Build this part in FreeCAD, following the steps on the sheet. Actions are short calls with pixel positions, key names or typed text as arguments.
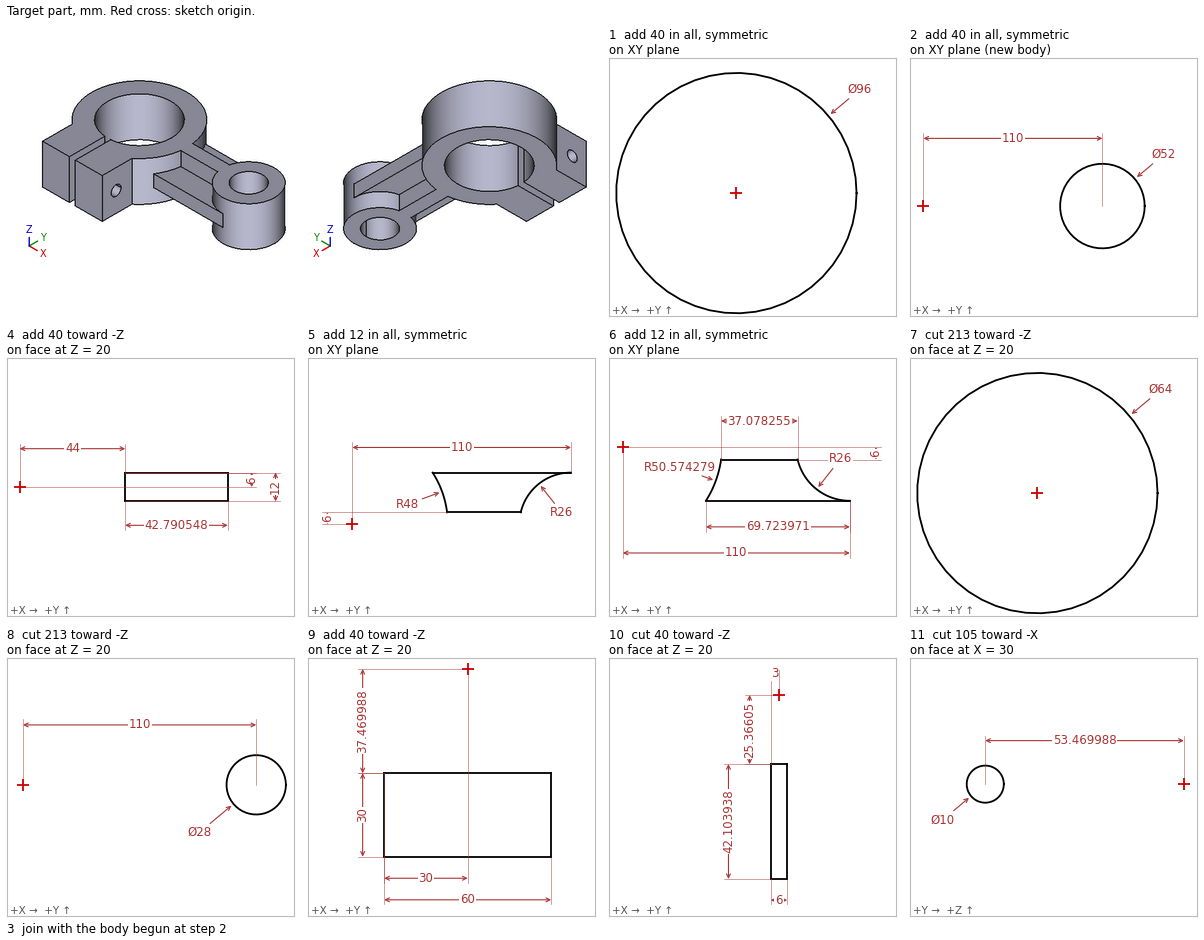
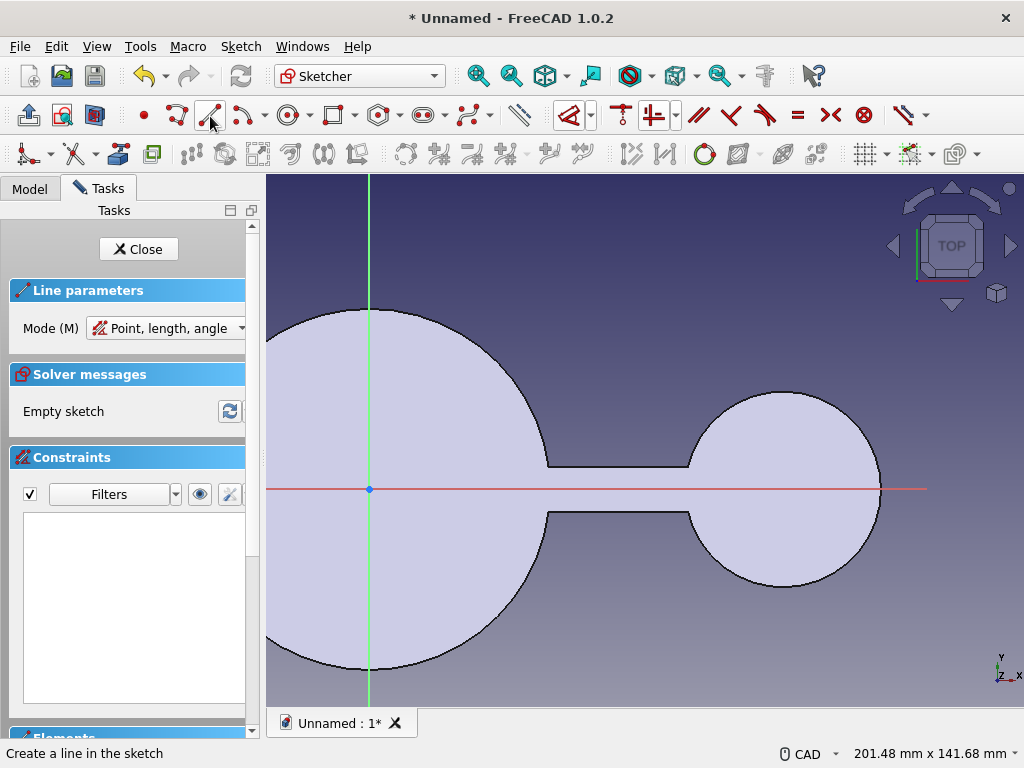
click(783, 392)
click(521, 392)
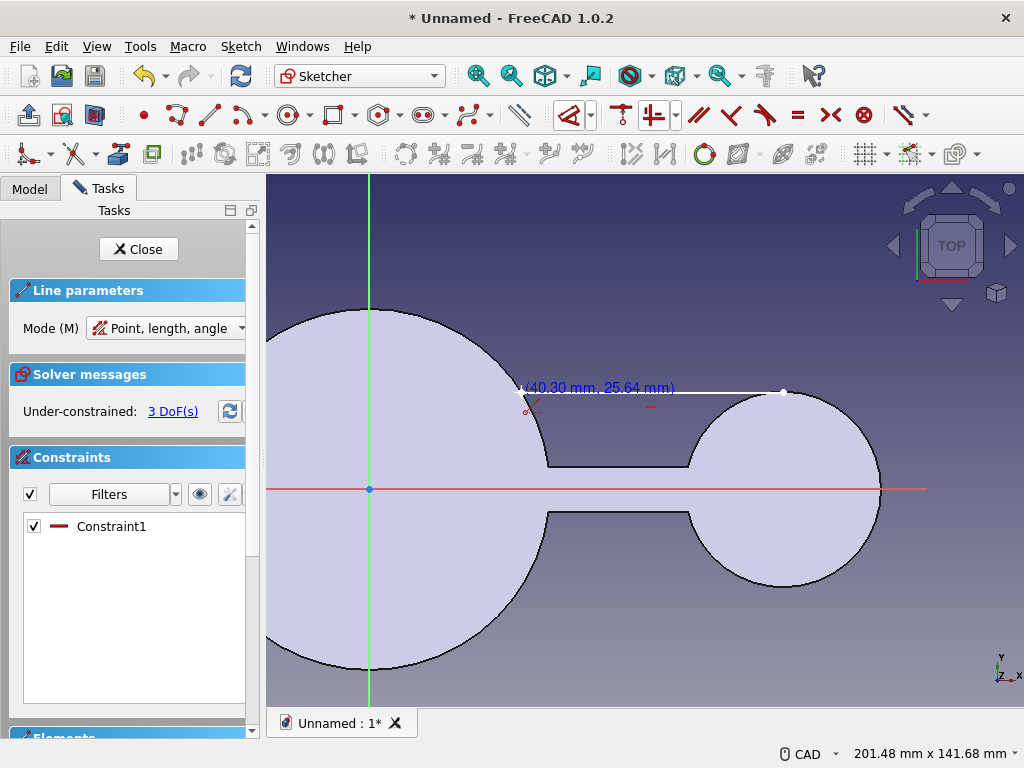
click(549, 467)
click(688, 467)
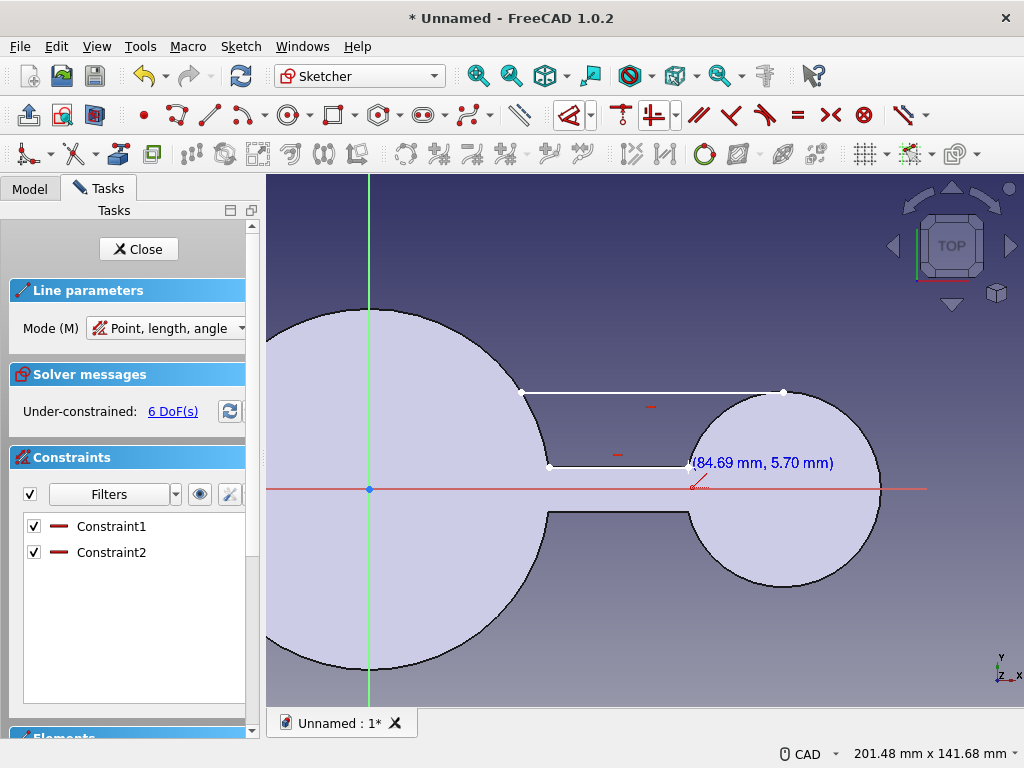
key(g)
key(3)
key(a)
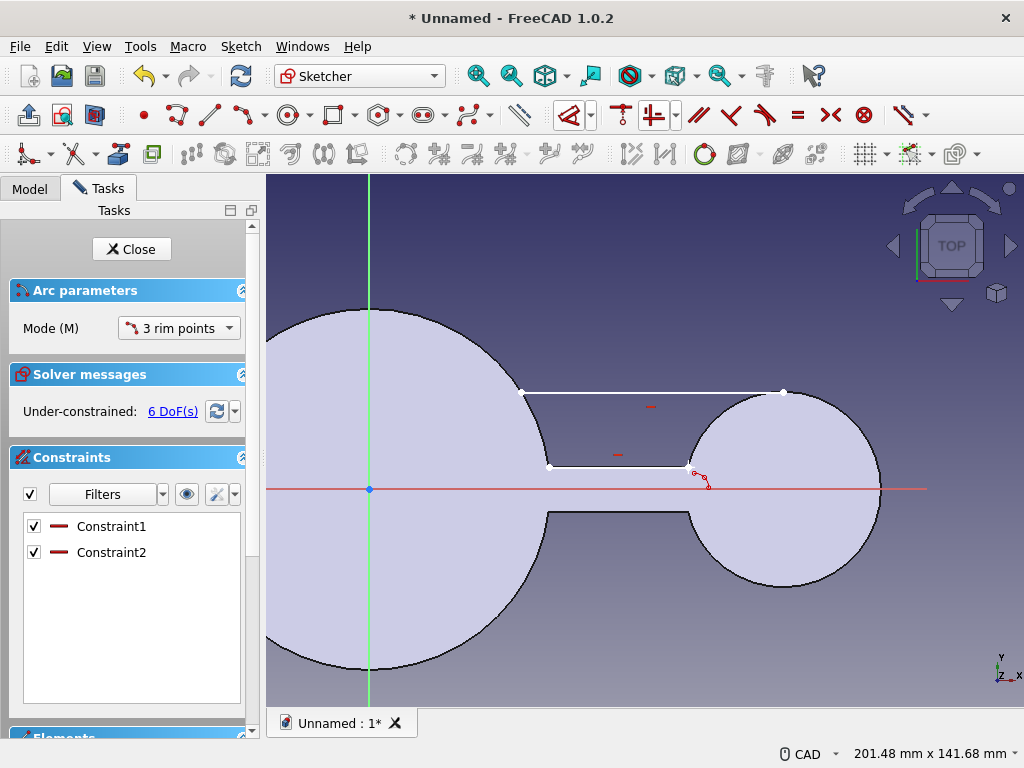
click(521, 393)
click(549, 468)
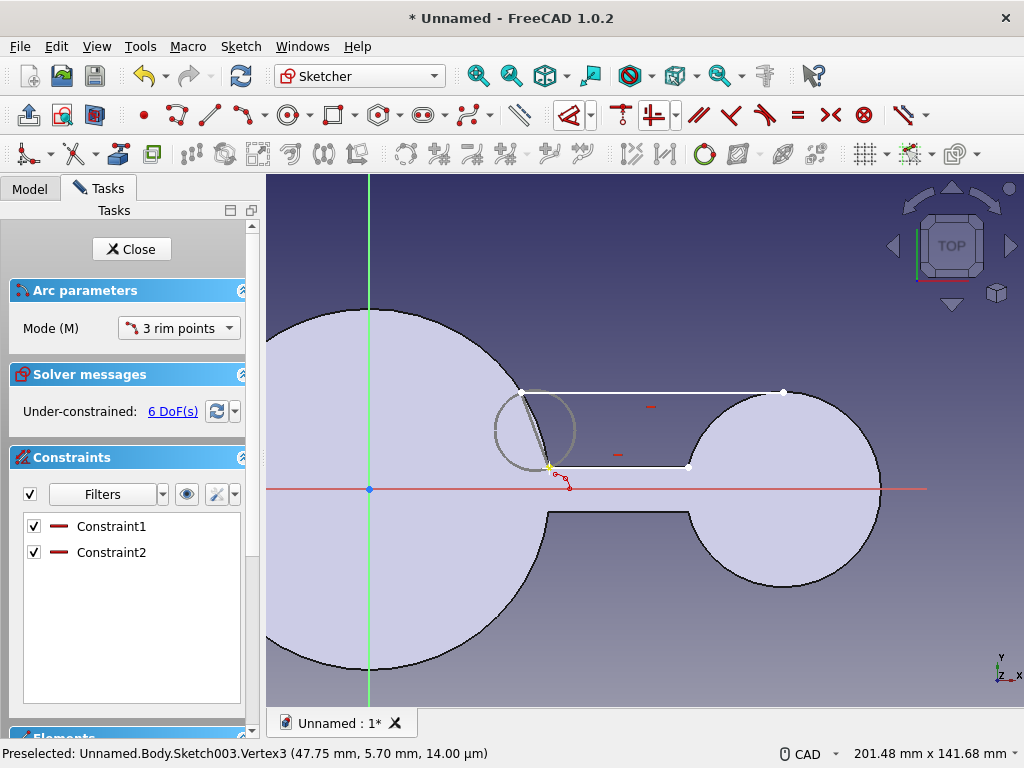
scroll(539, 428, up, 7)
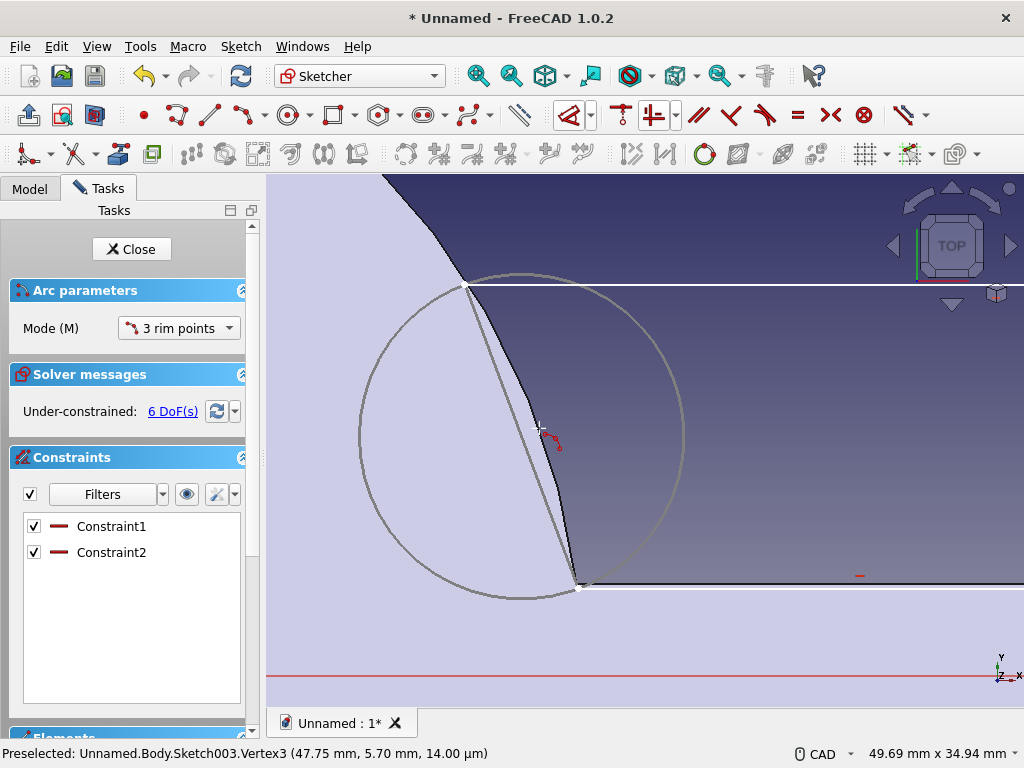
click(538, 425)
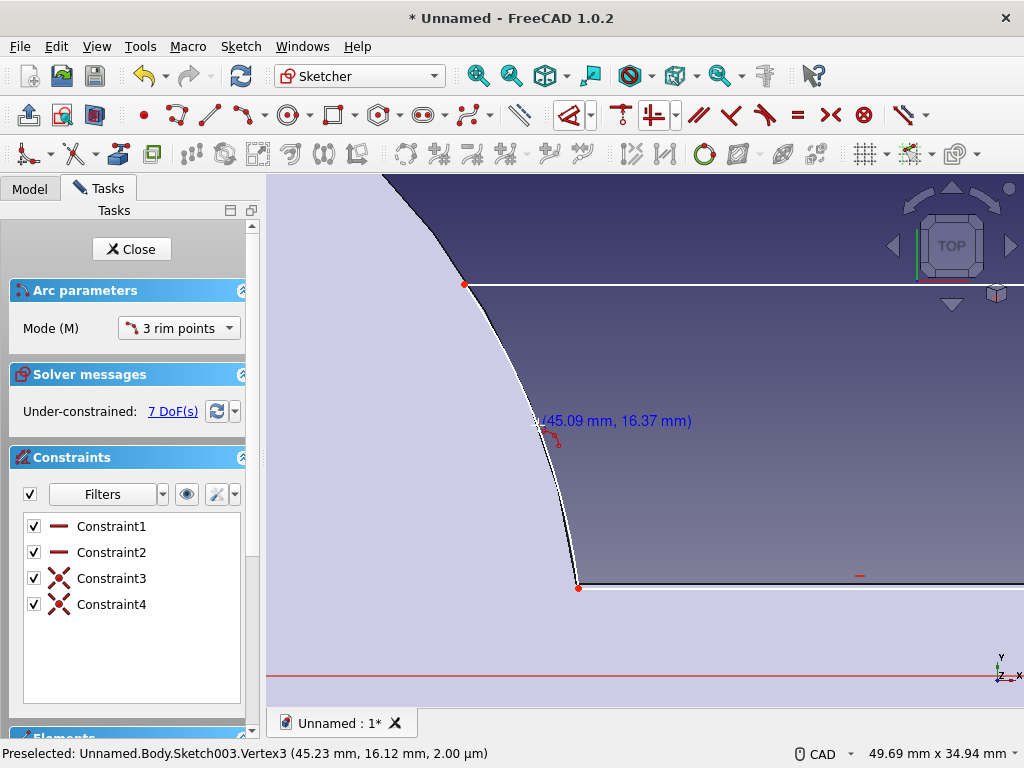
scroll(540, 428, down, 7)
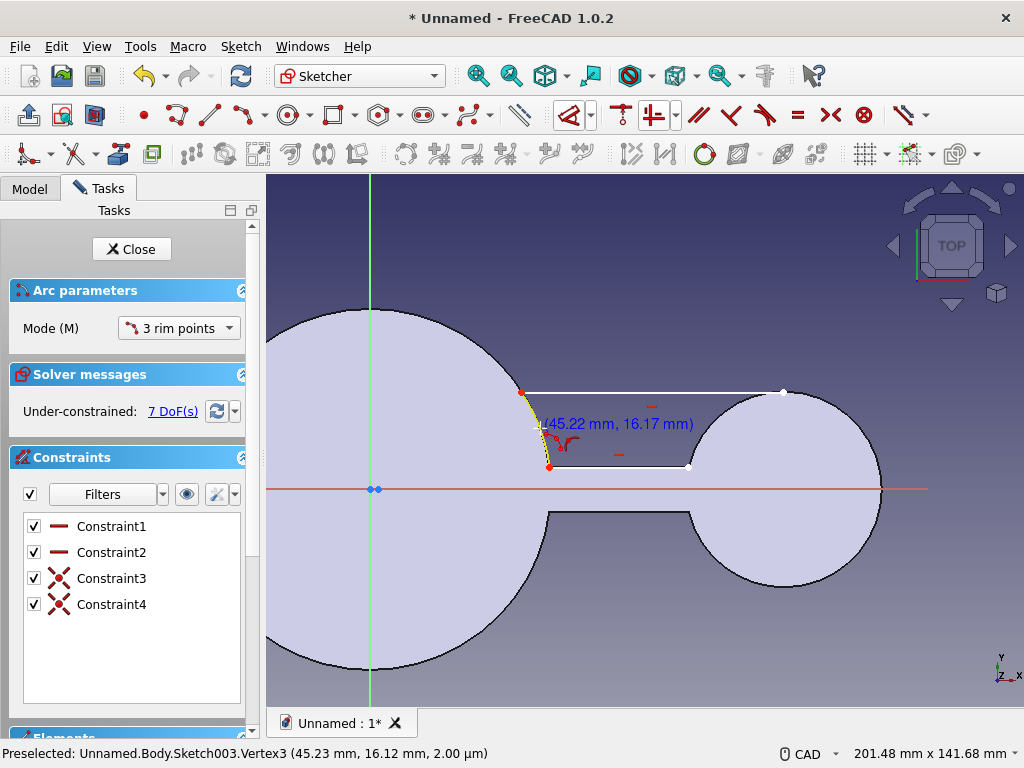
click(689, 468)
click(784, 393)
click(723, 413)
key(Escape)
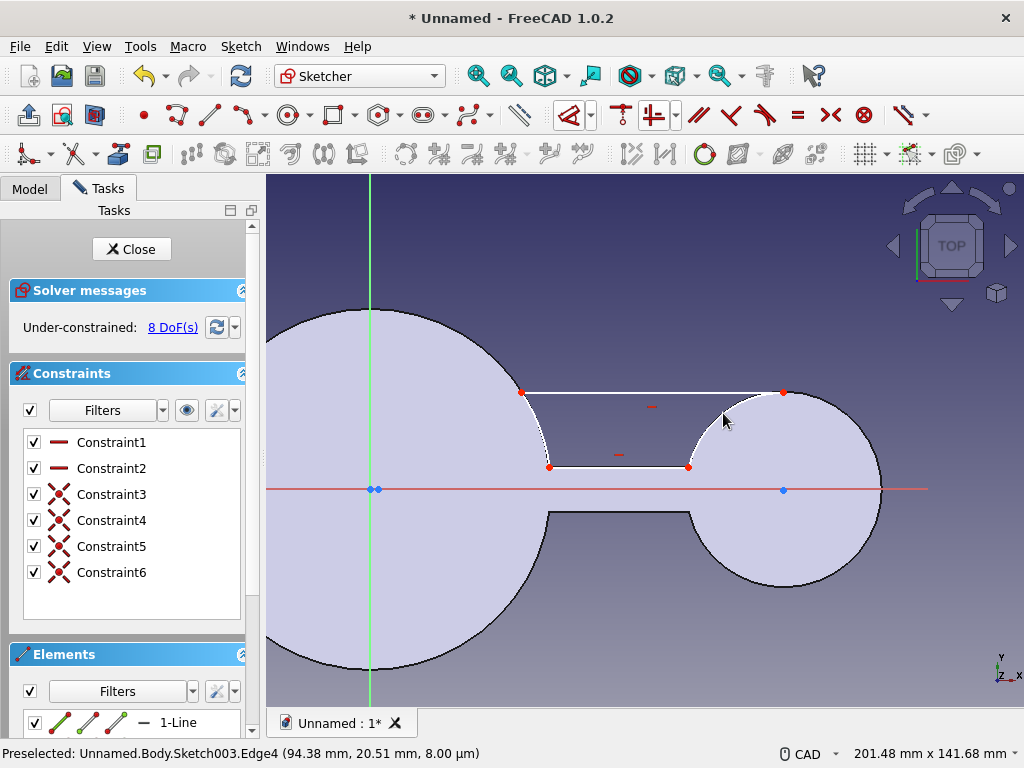
click(705, 393)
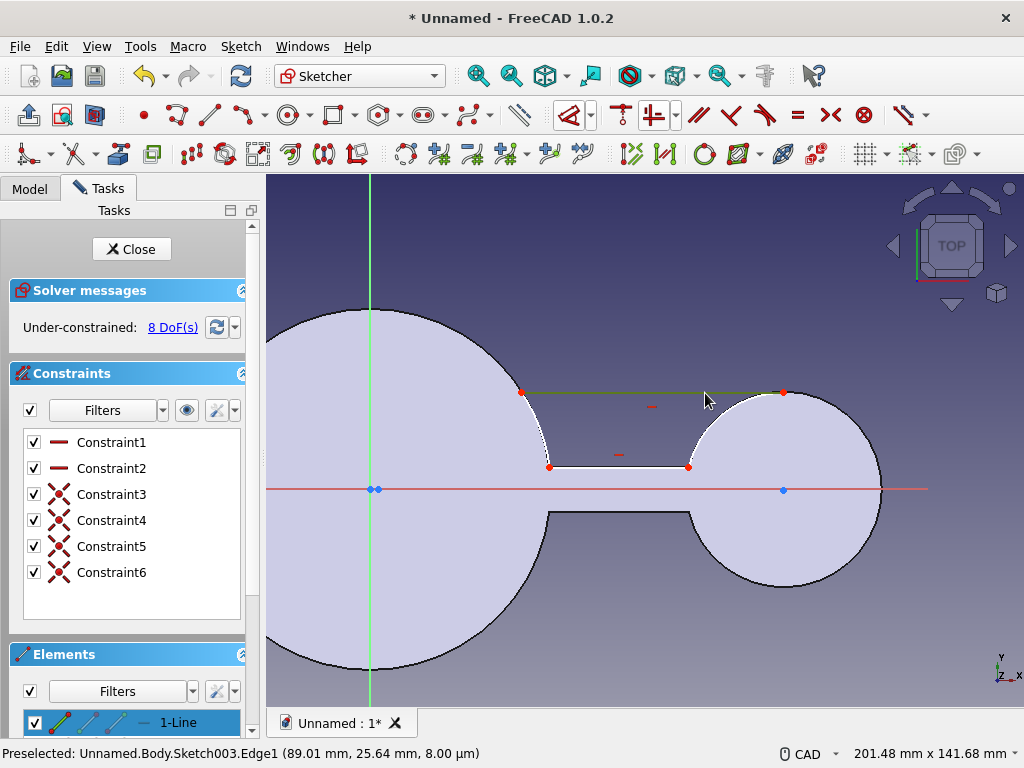
click(705, 433)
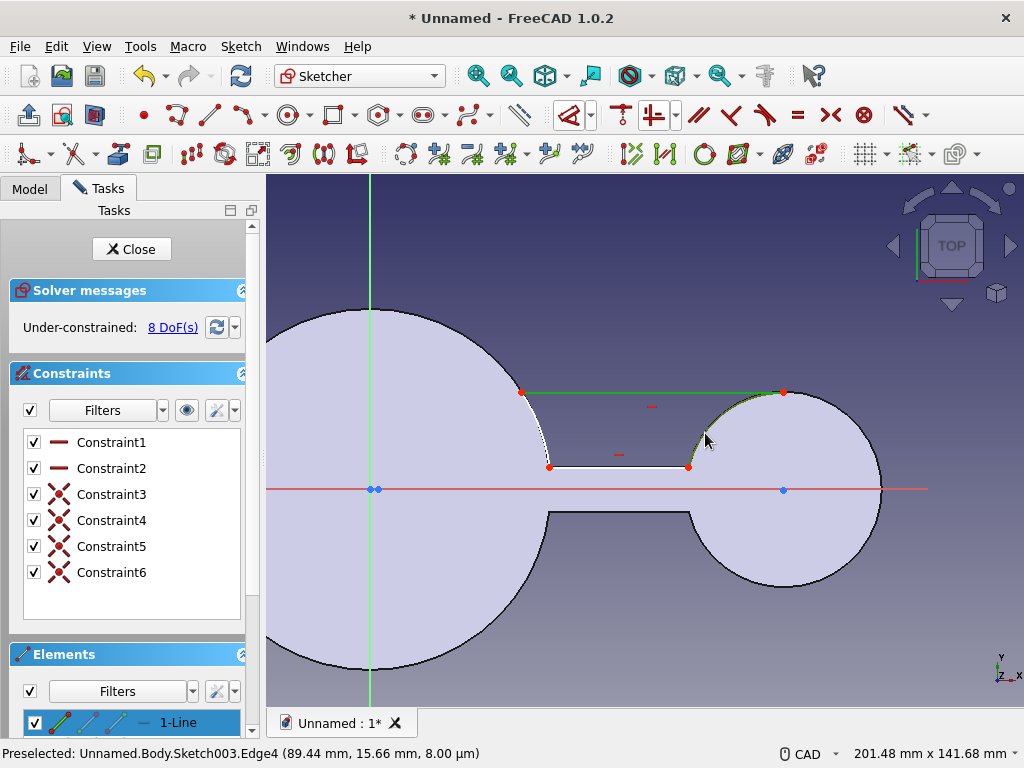
click(765, 116)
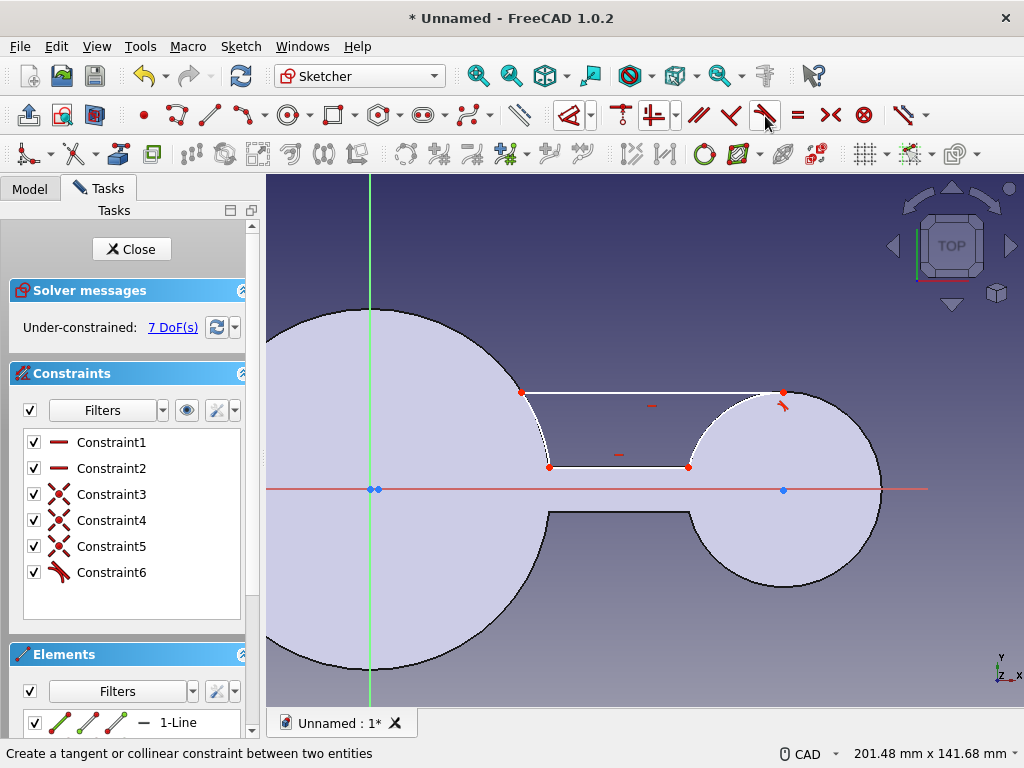
drag(360, 479, 388, 499)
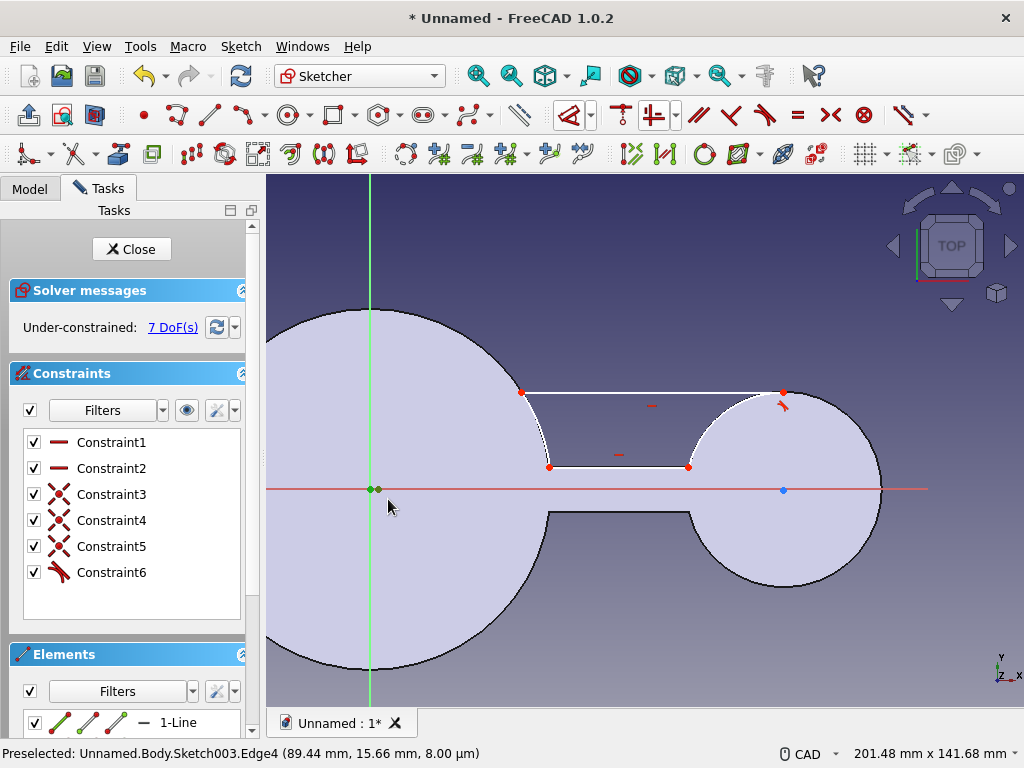
click(621, 116)